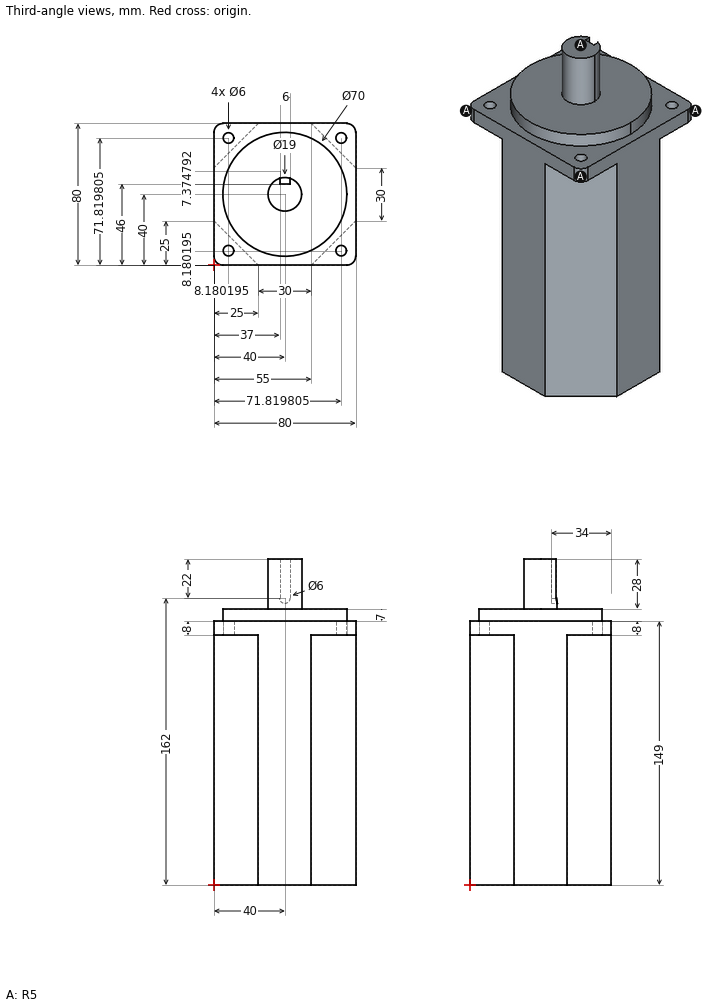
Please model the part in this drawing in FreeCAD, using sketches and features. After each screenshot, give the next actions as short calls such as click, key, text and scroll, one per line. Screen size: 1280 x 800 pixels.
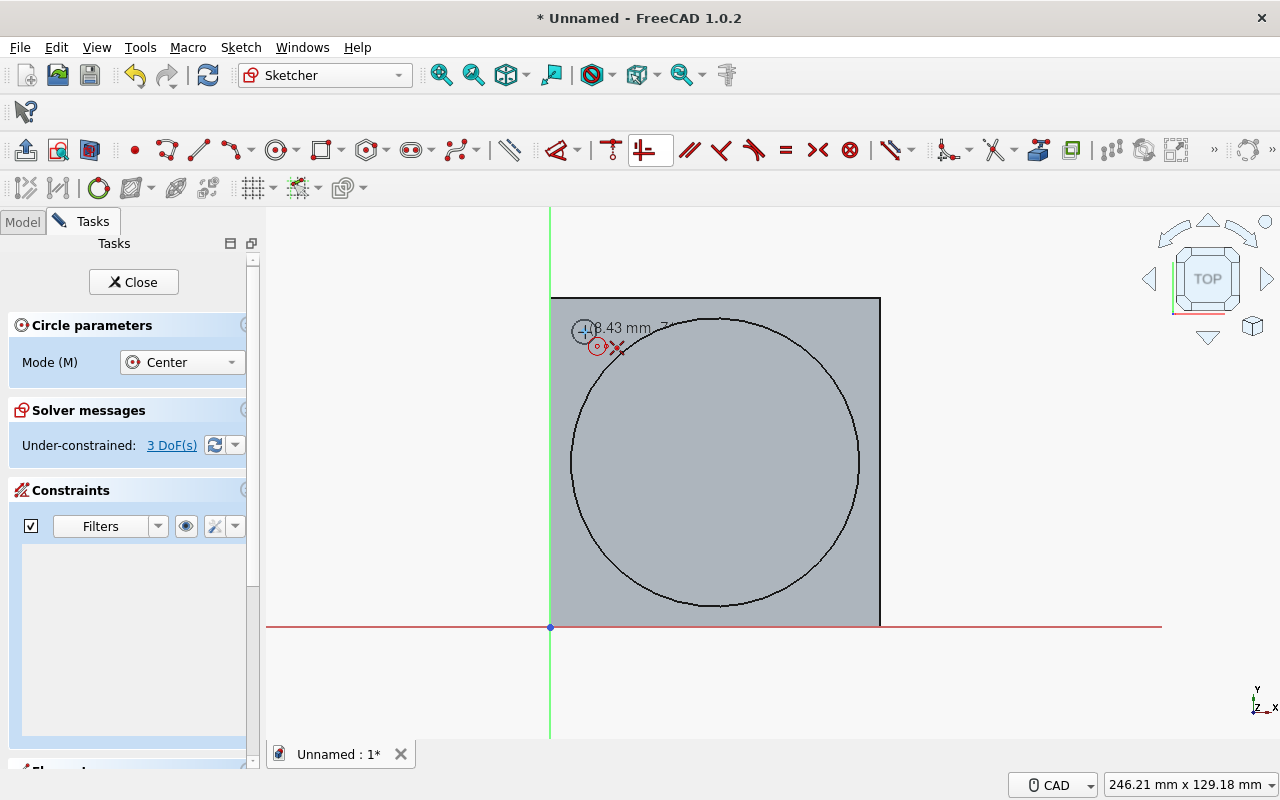
scroll(846, 331, up, 4)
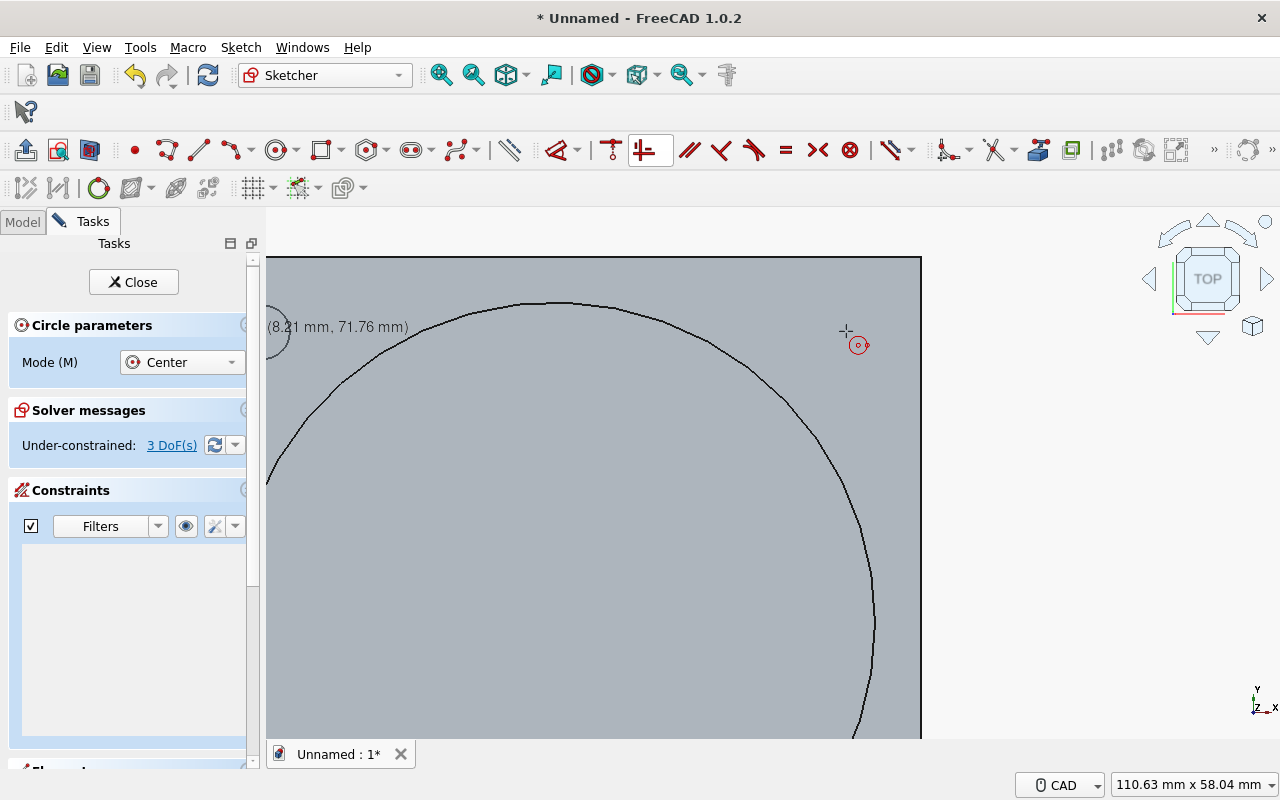
click(846, 332)
click(865, 312)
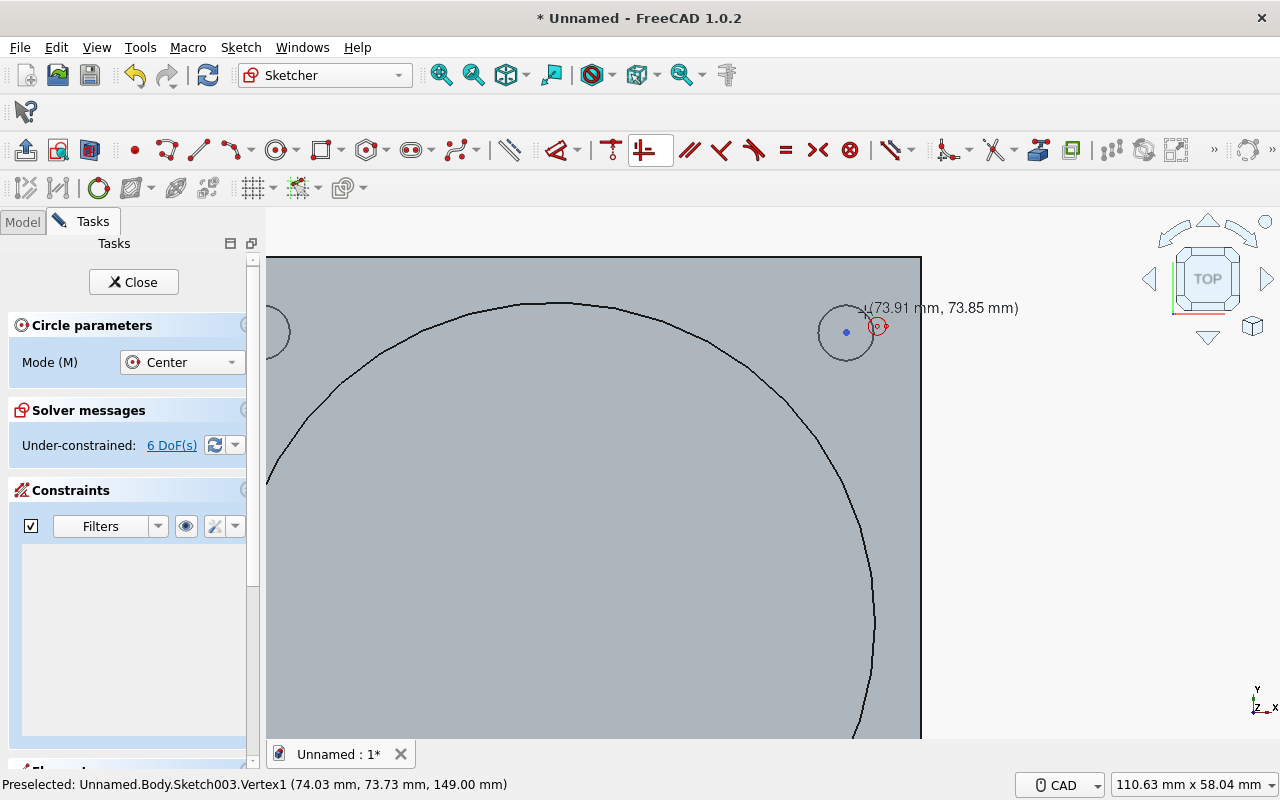
scroll(846, 331, down, 4)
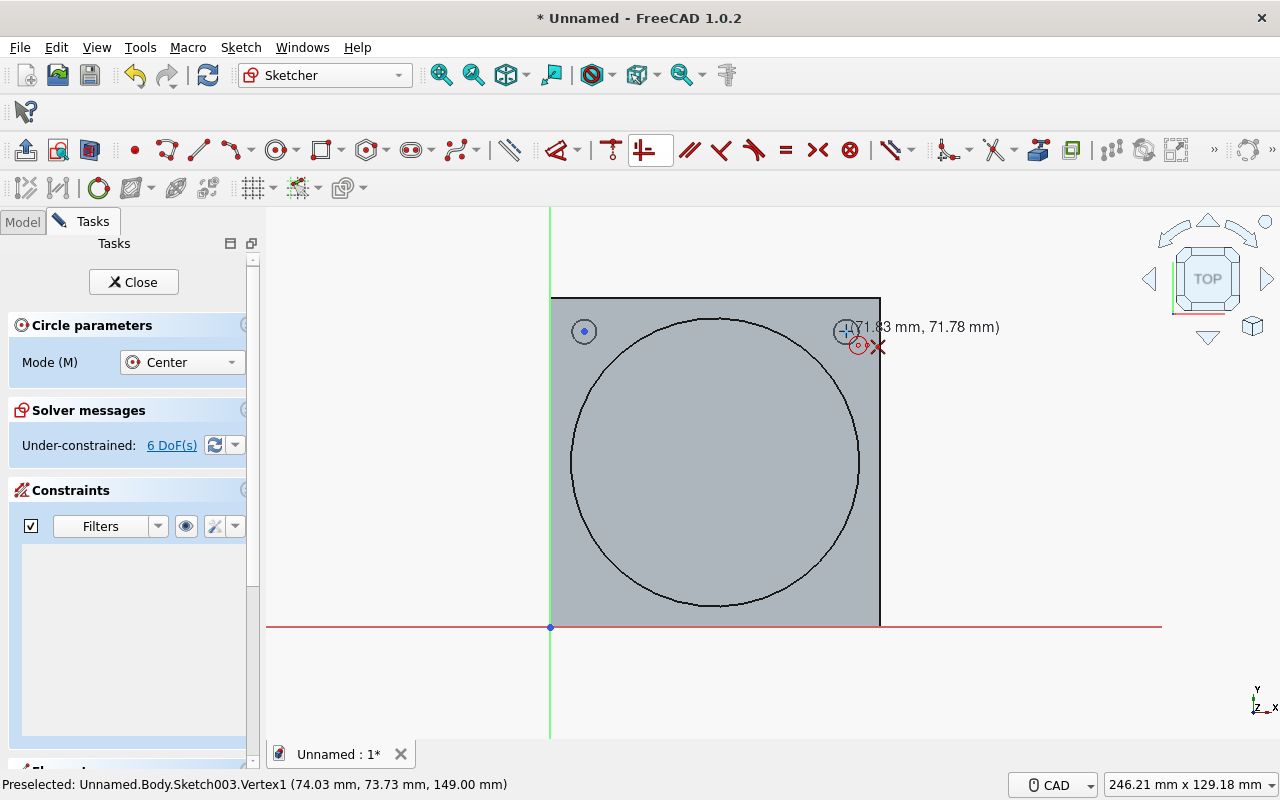
scroll(846, 594, up, 4)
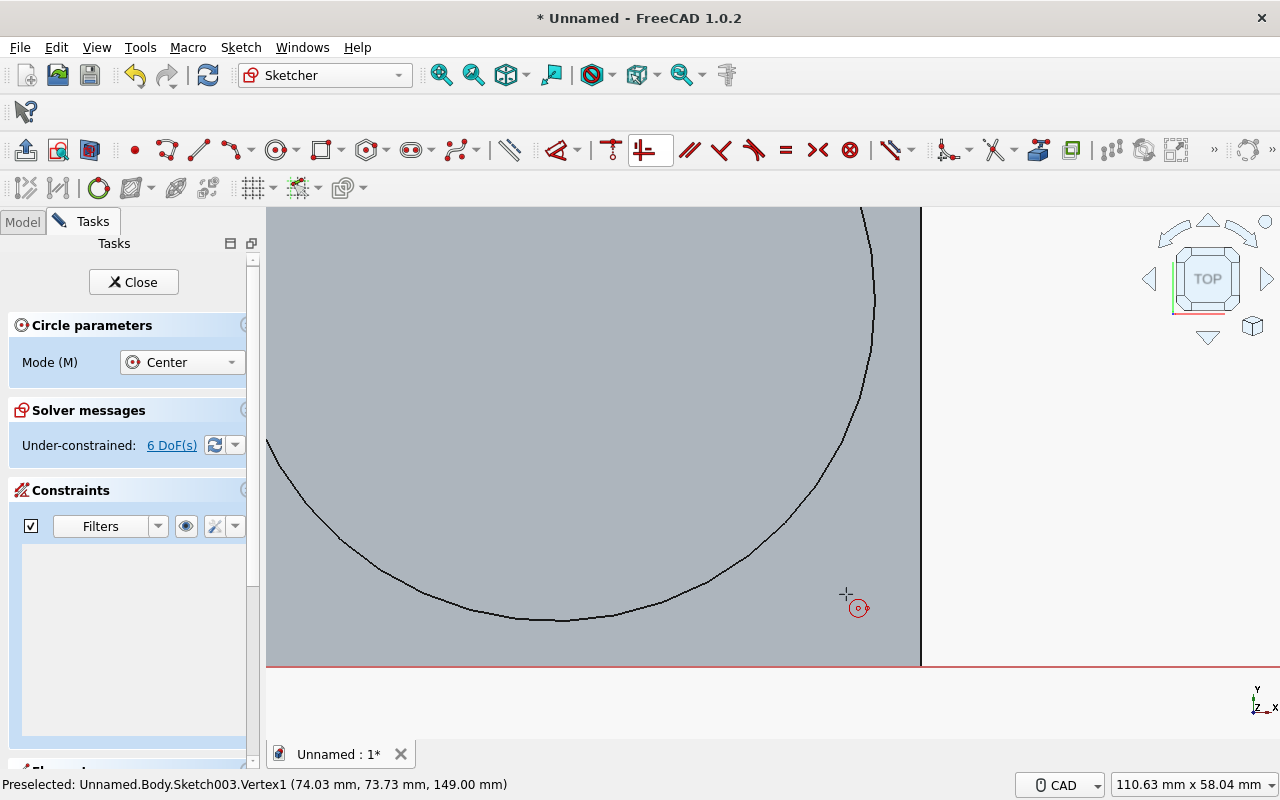
click(846, 592)
click(865, 573)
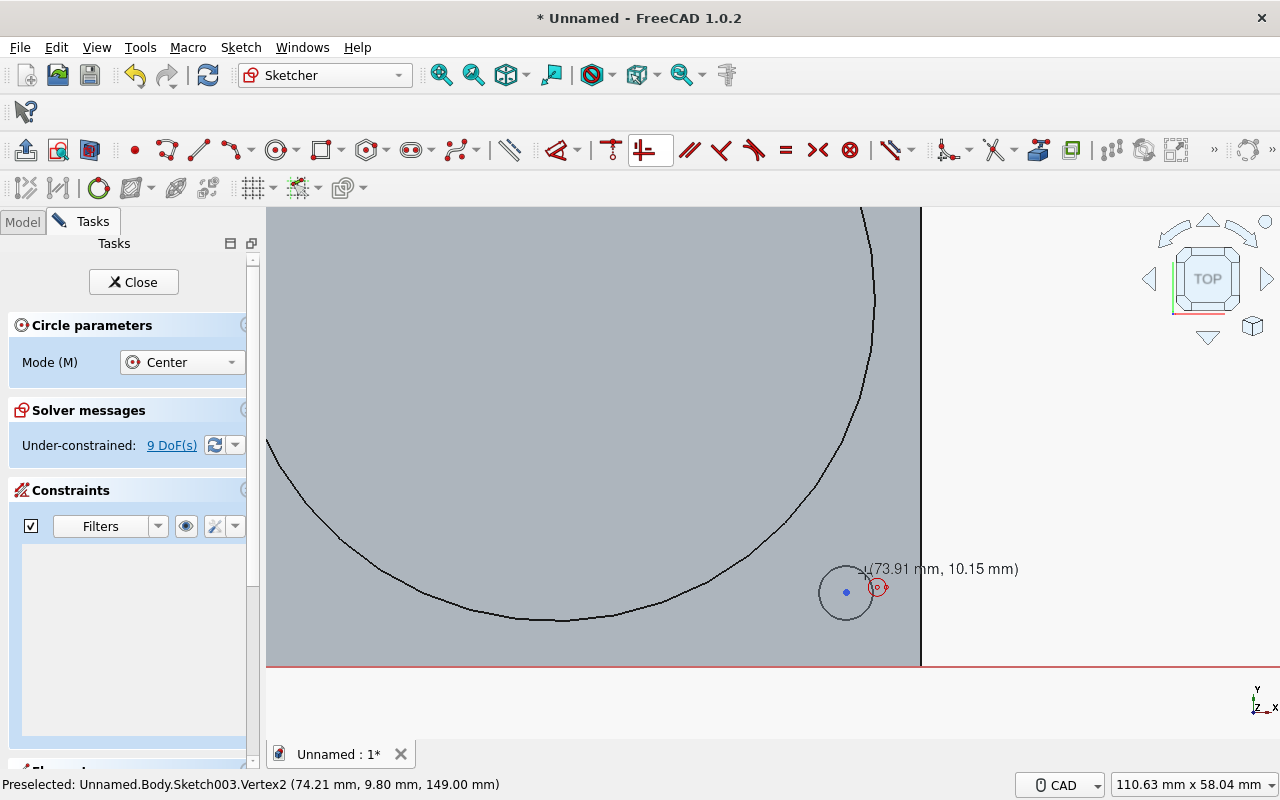
scroll(846, 594, down, 4)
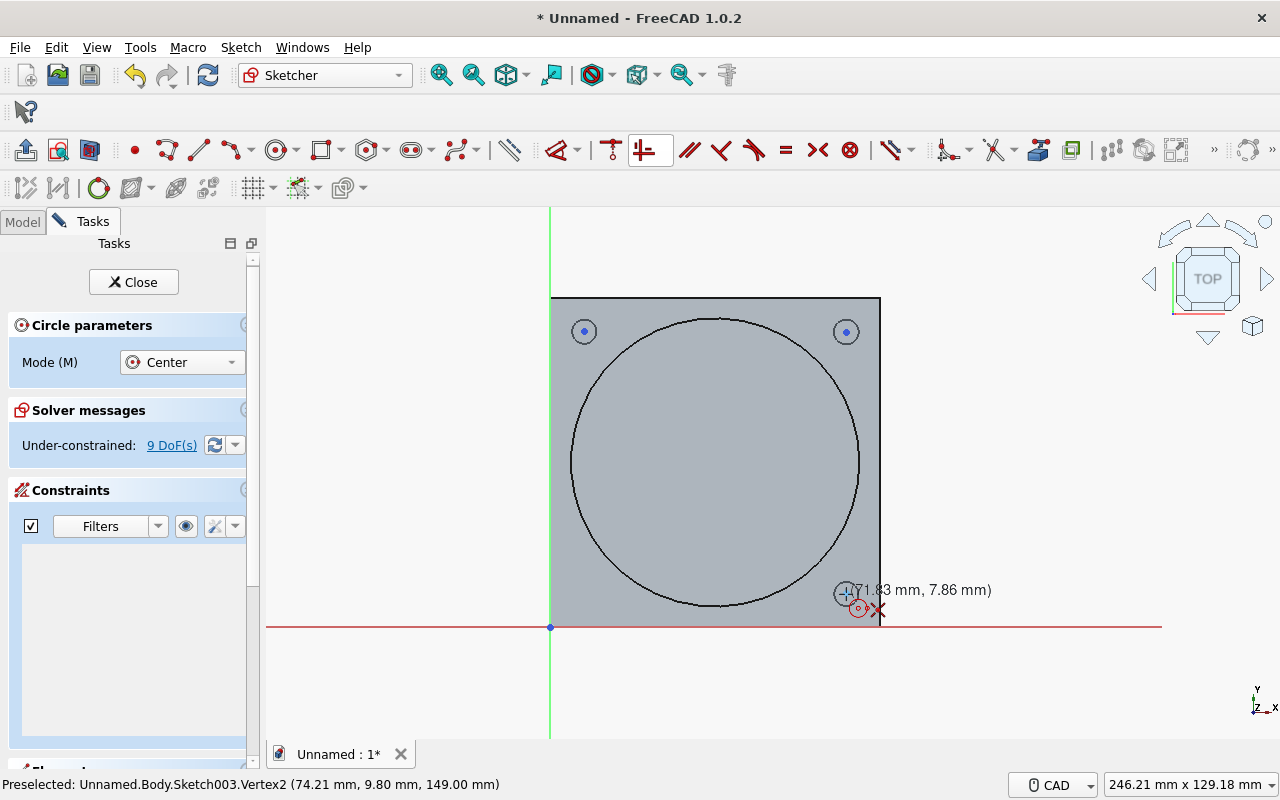
scroll(584, 594, up, 4)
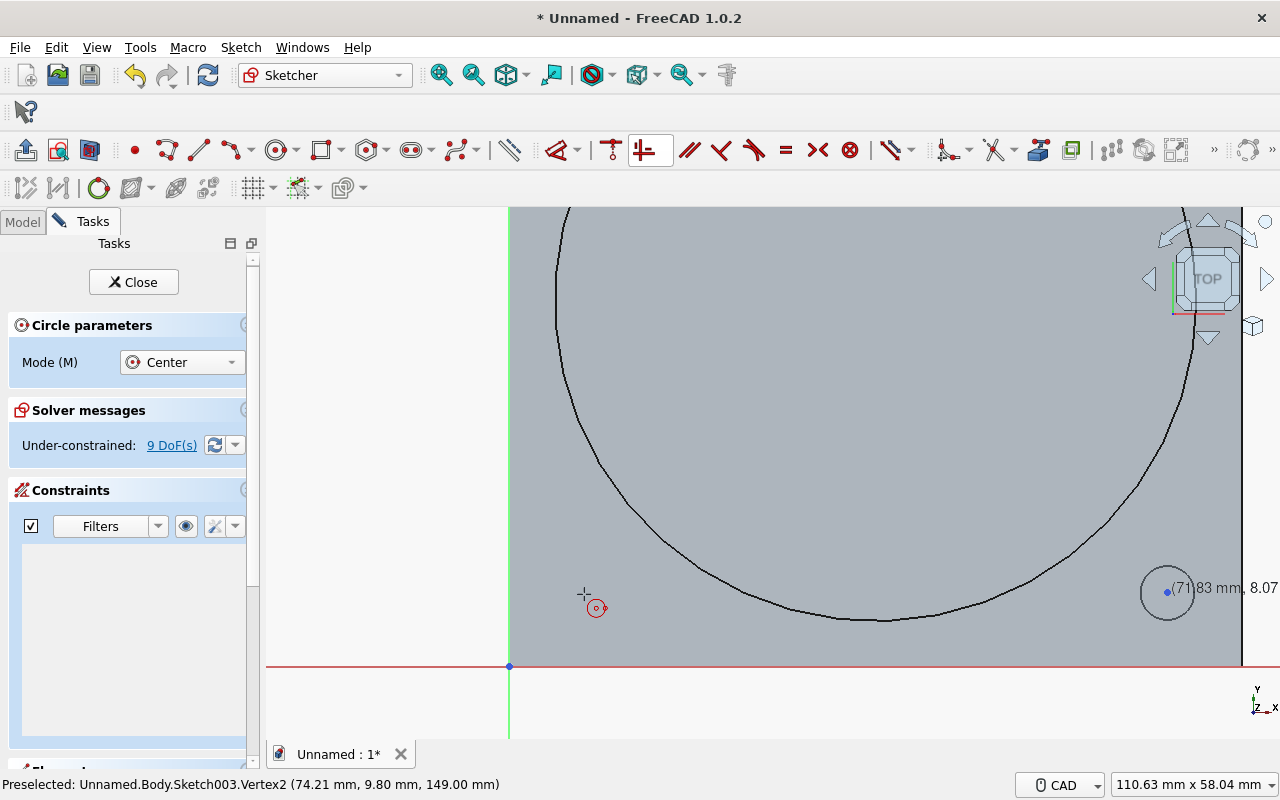
click(584, 592)
click(603, 573)
key(Escape)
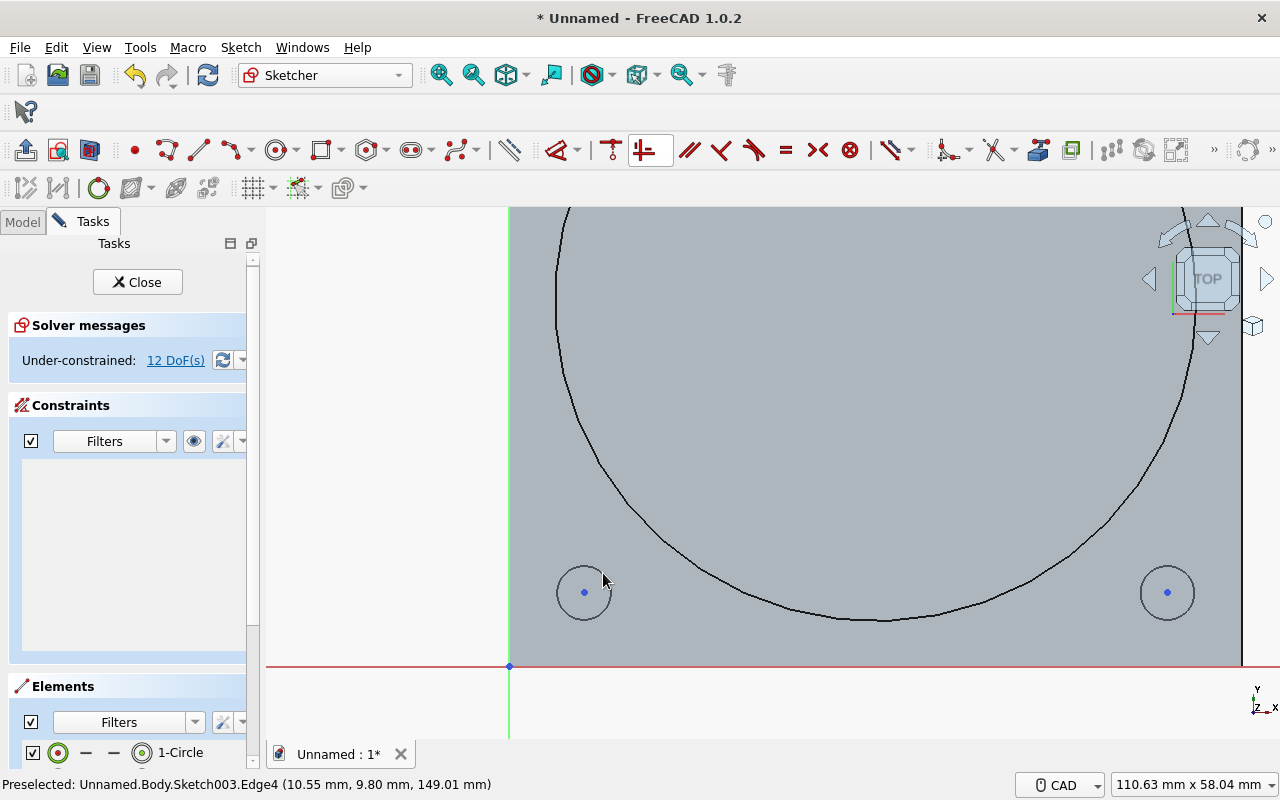
scroll(584, 594, down, 4)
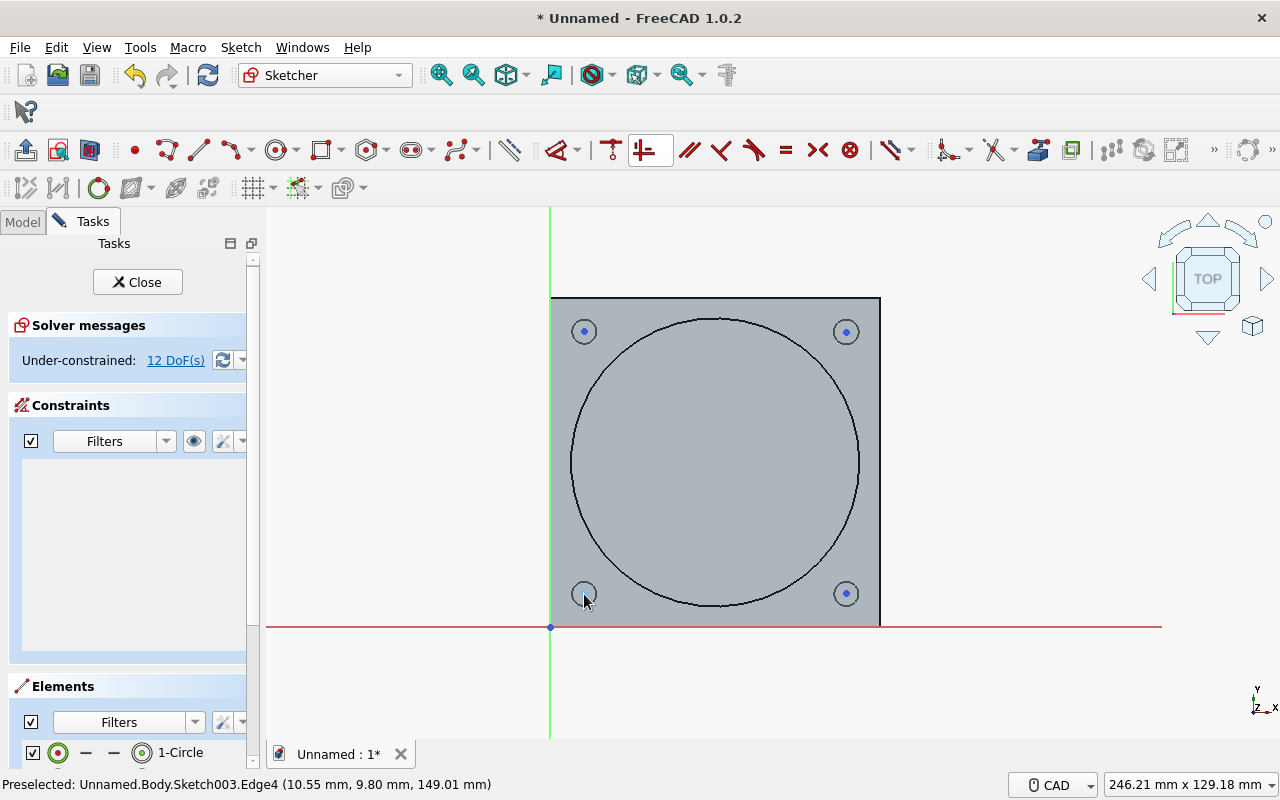
click(593, 323)